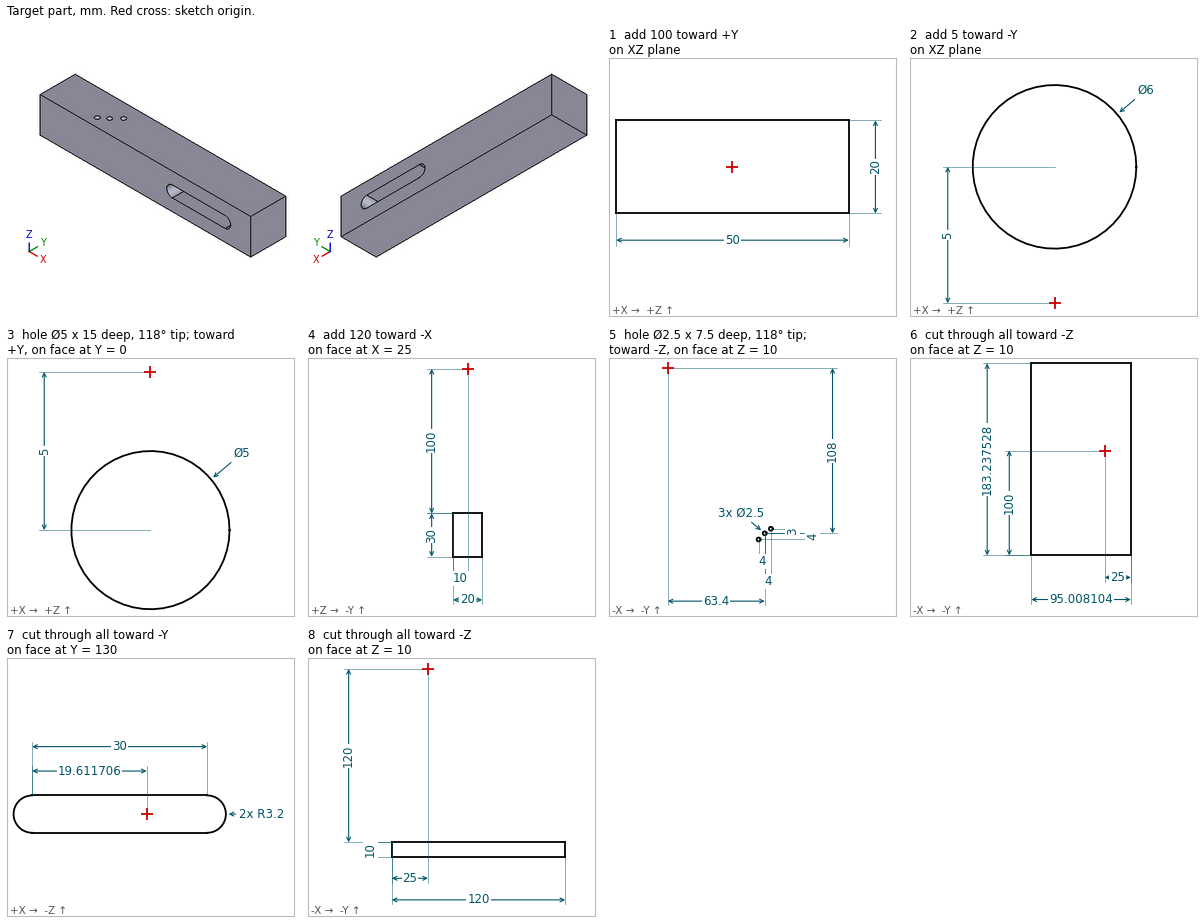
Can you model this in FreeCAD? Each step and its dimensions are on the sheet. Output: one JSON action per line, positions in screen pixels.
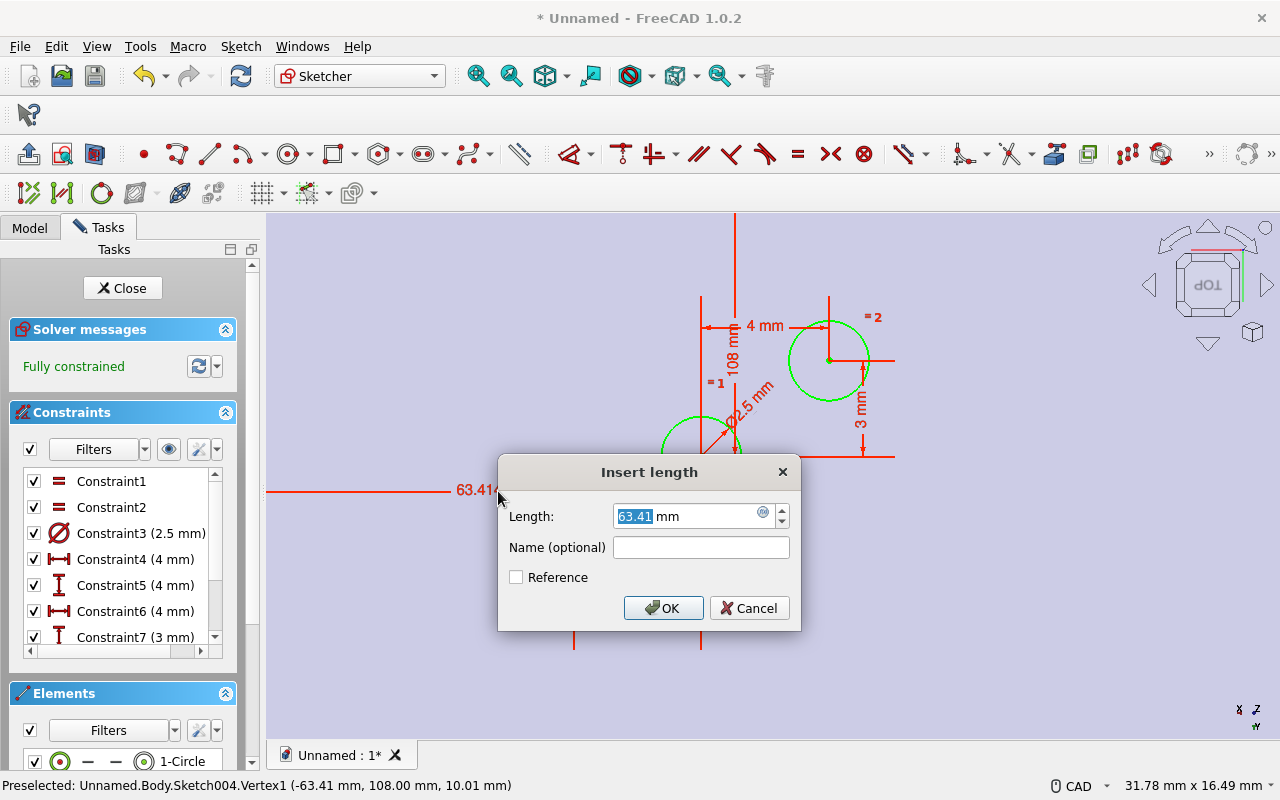
{"action": "type", "text": "63.4"}
{"action": "key", "text": "Return"}
{"action": "key", "text": "Escape"}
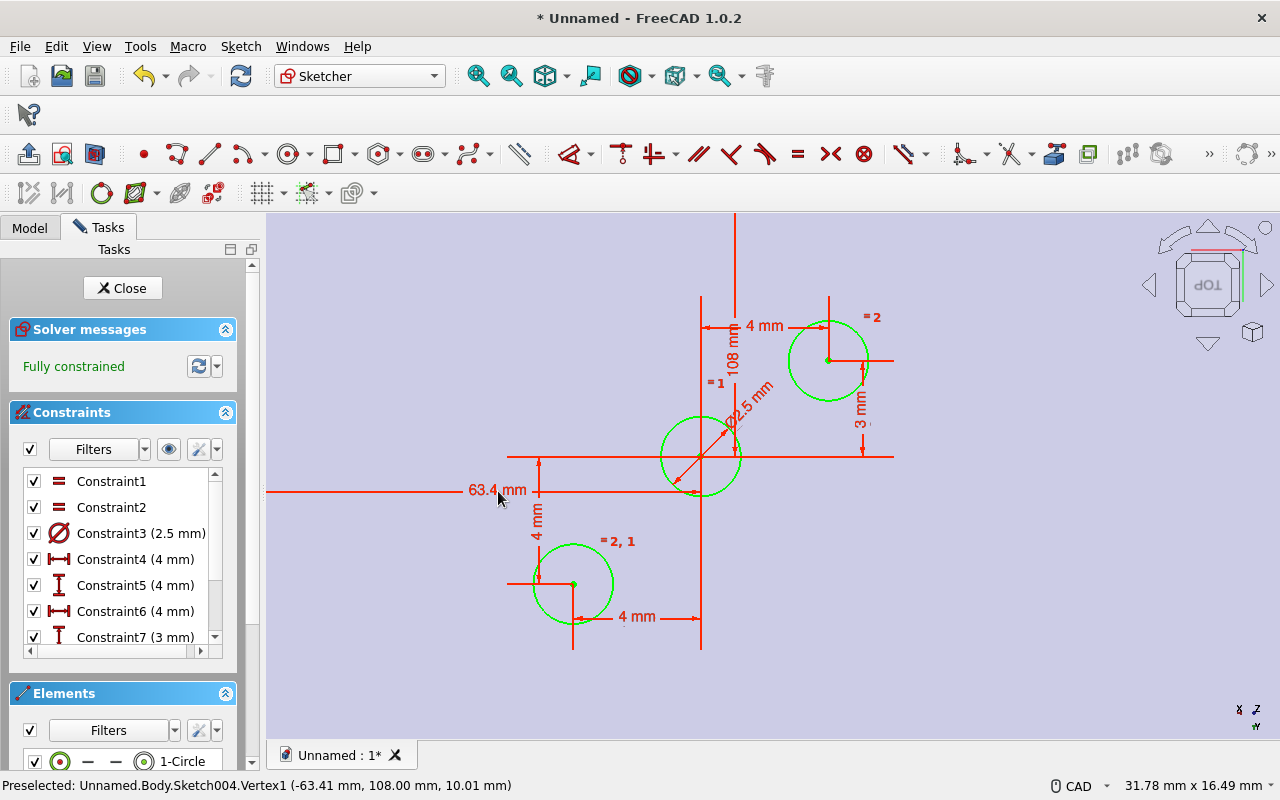
{"action": "left_click", "coordinate": [123, 288]}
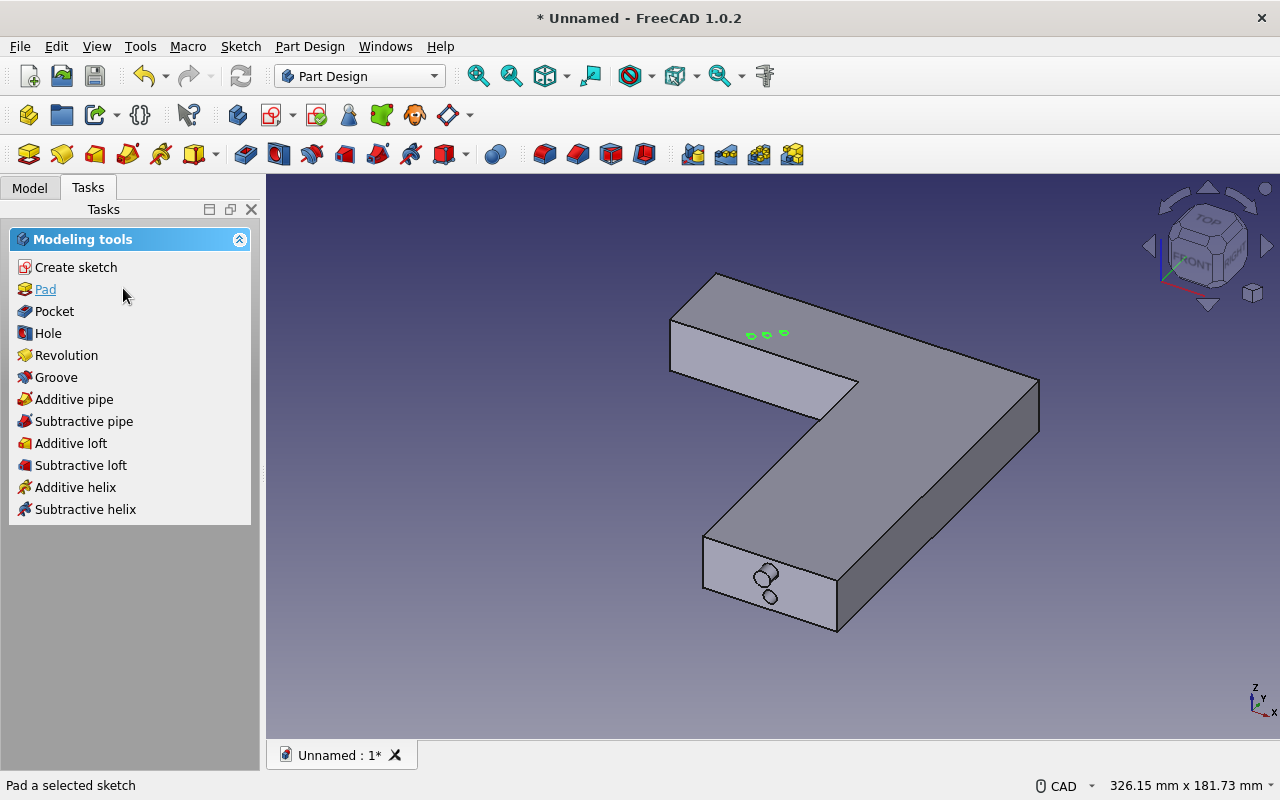
{"action": "left_click", "coordinate": [279, 154]}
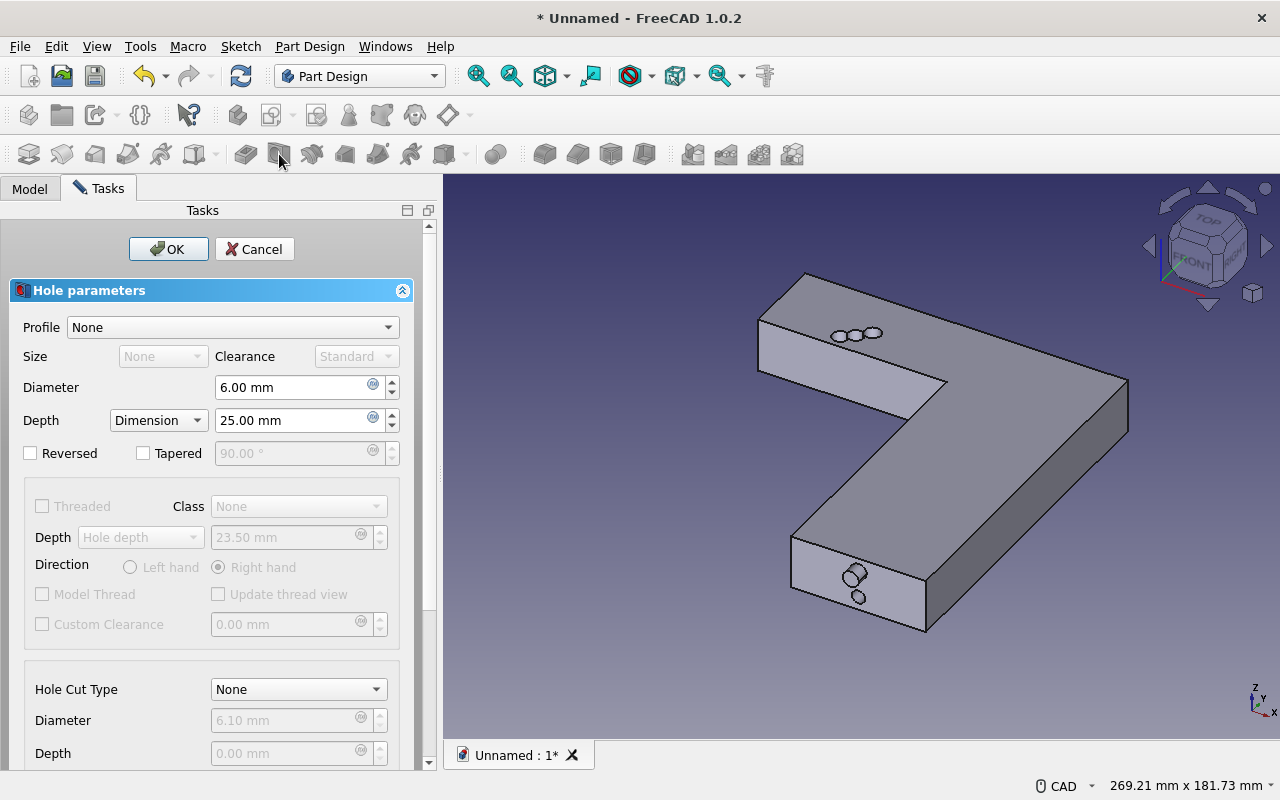
{"action": "triple_click", "coordinate": [300, 388]}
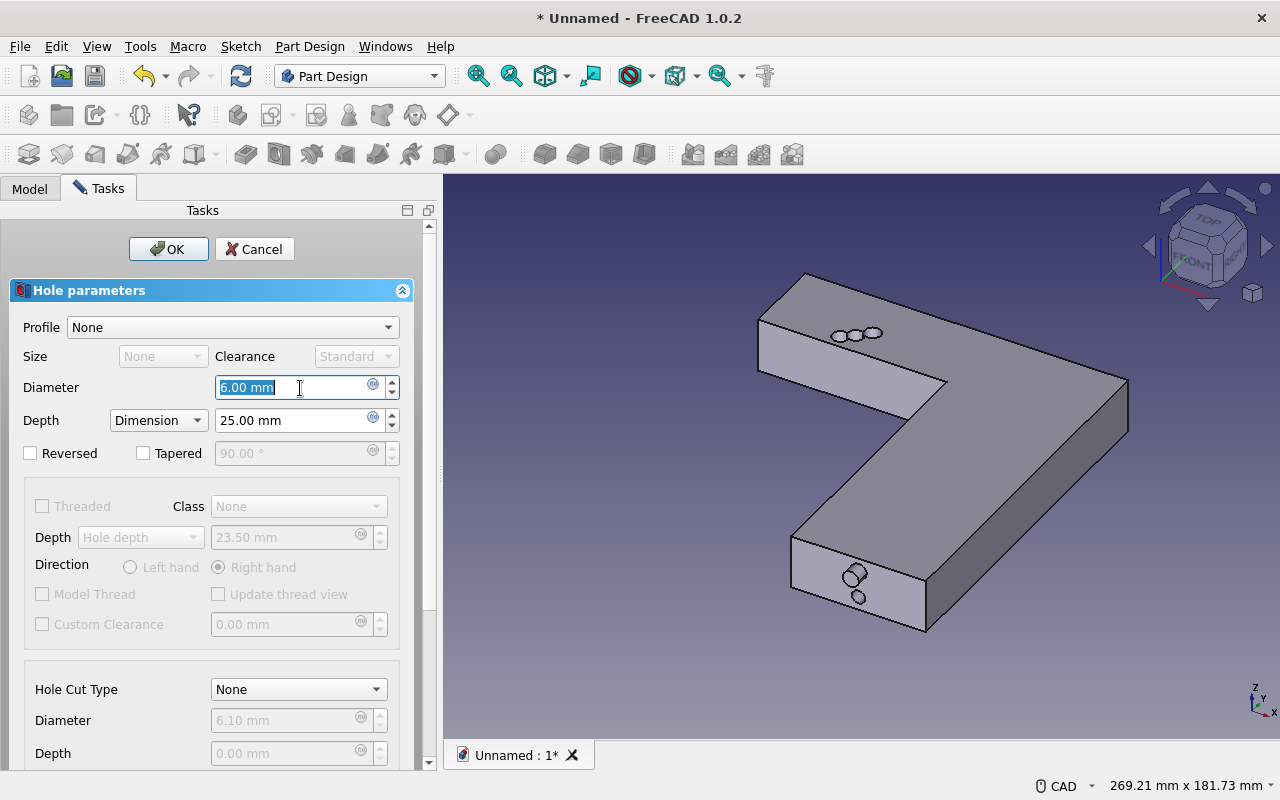
{"action": "type", "text": "2.5"}
{"action": "key", "text": "Tab"}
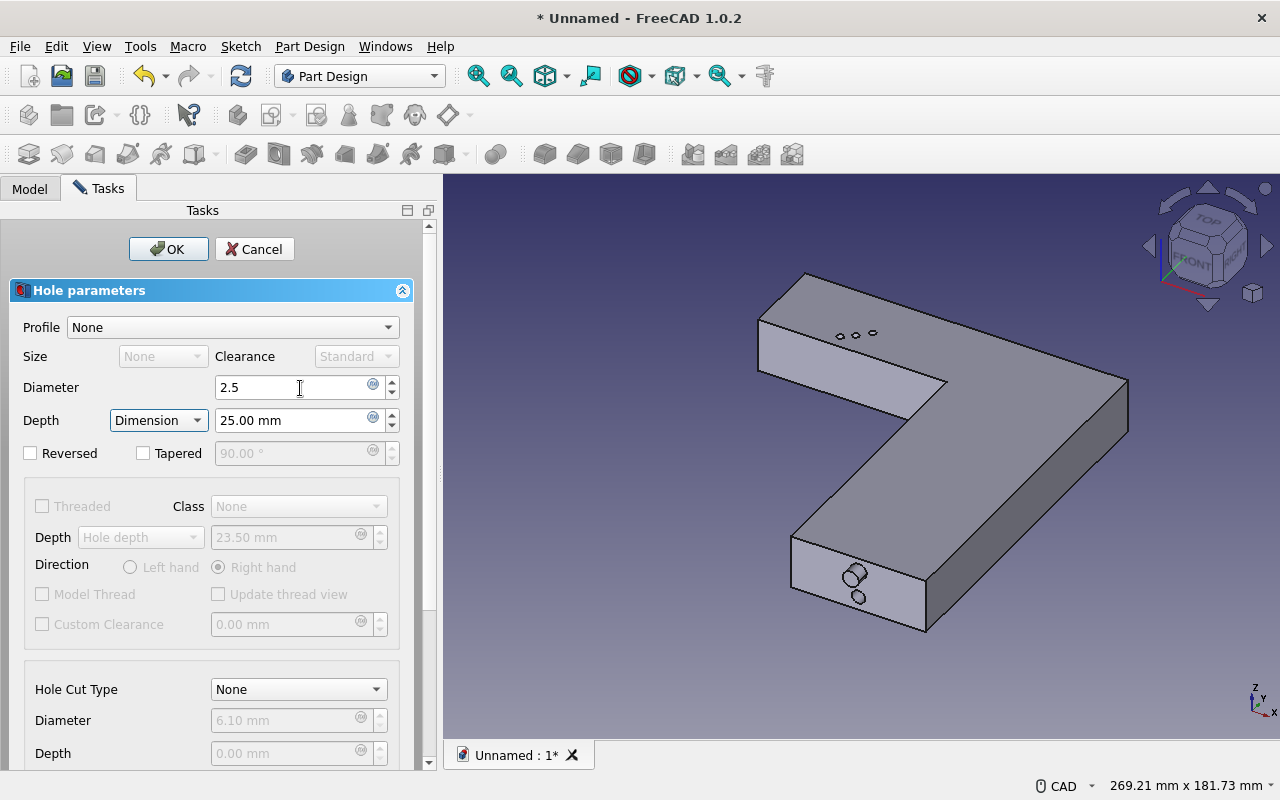
{"action": "triple_click", "coordinate": [300, 420]}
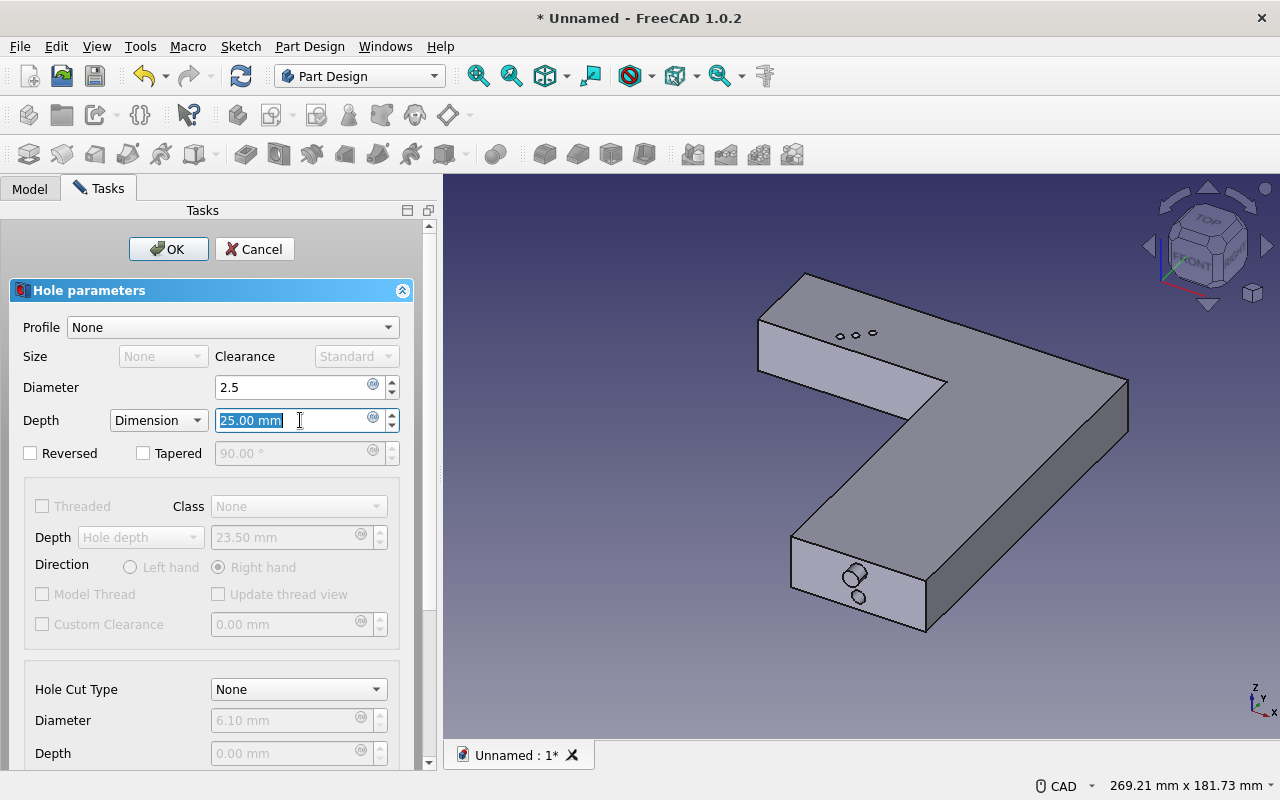
{"action": "type", "text": "7.5"}
{"action": "key", "text": "Tab"}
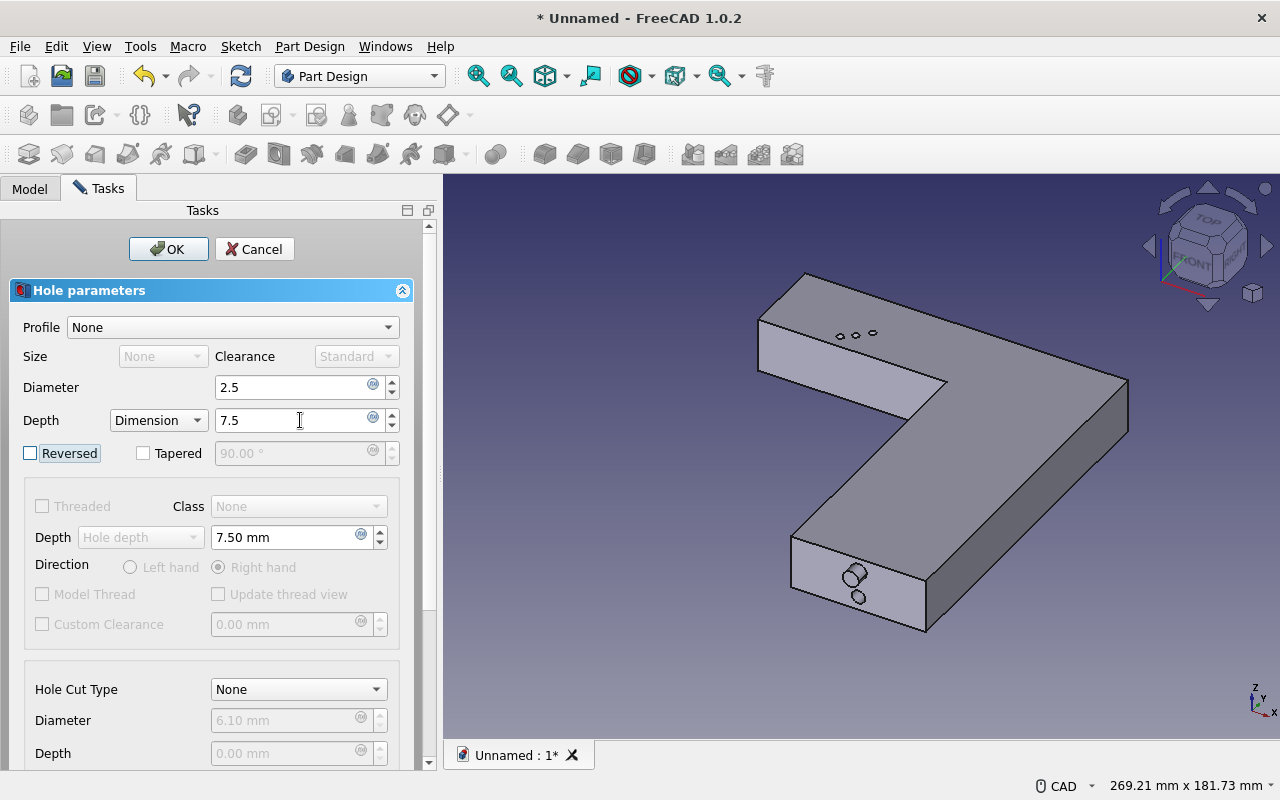
{"action": "left_click", "coordinate": [169, 249]}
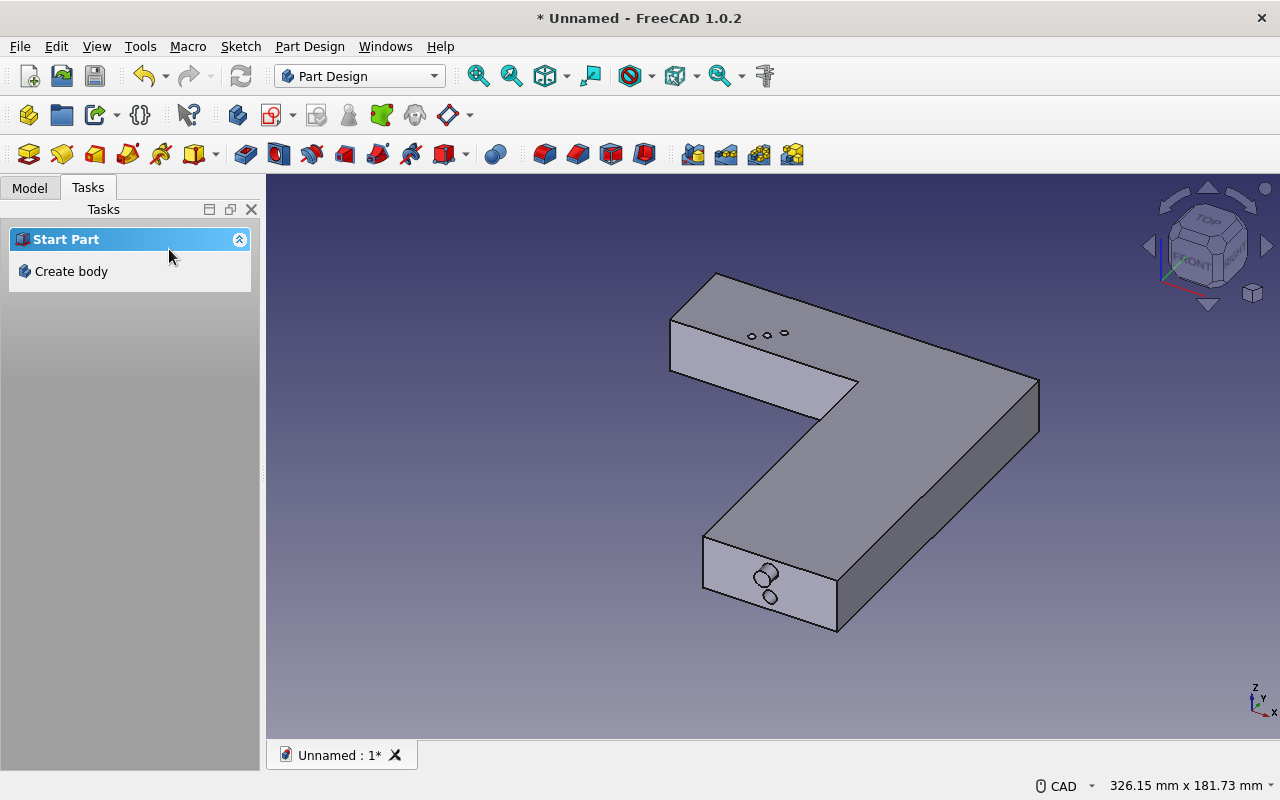
{"action": "left_click", "coordinate": [927, 399]}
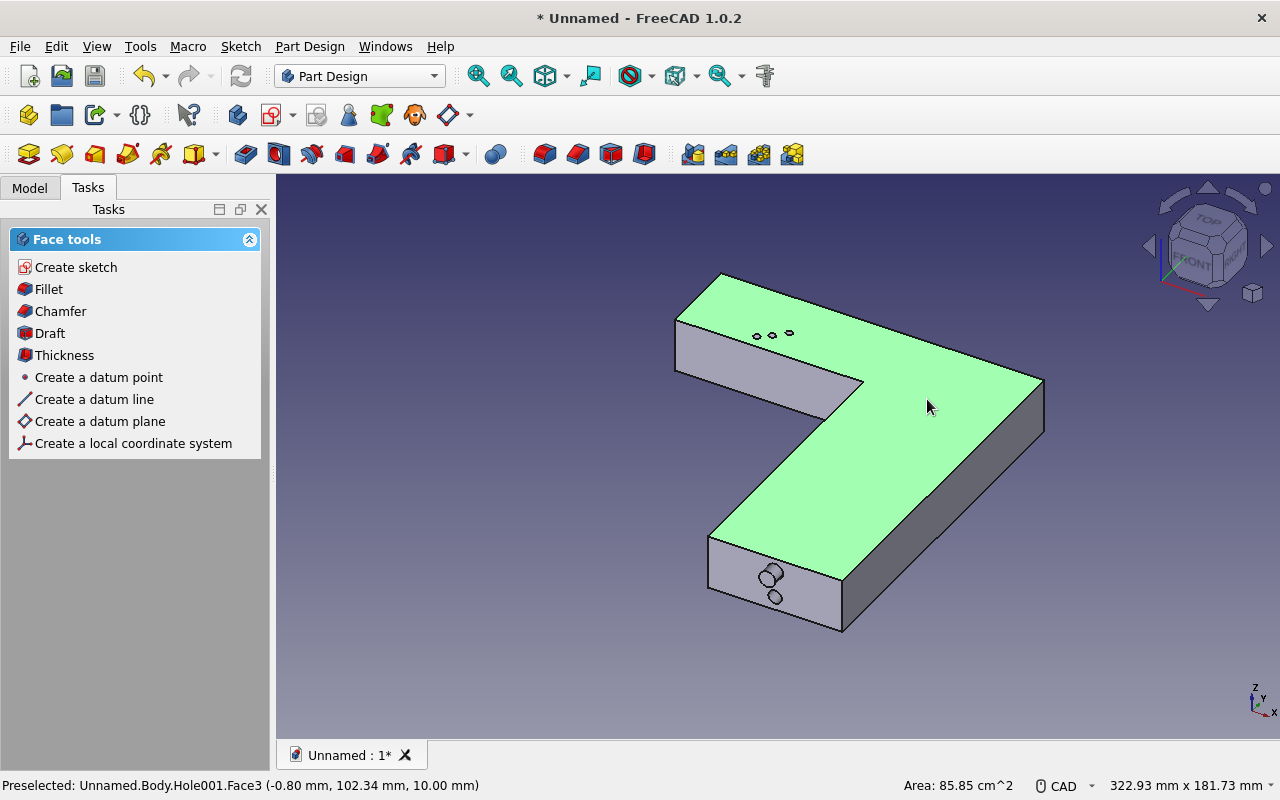
{"action": "left_click", "coordinate": [270, 116]}